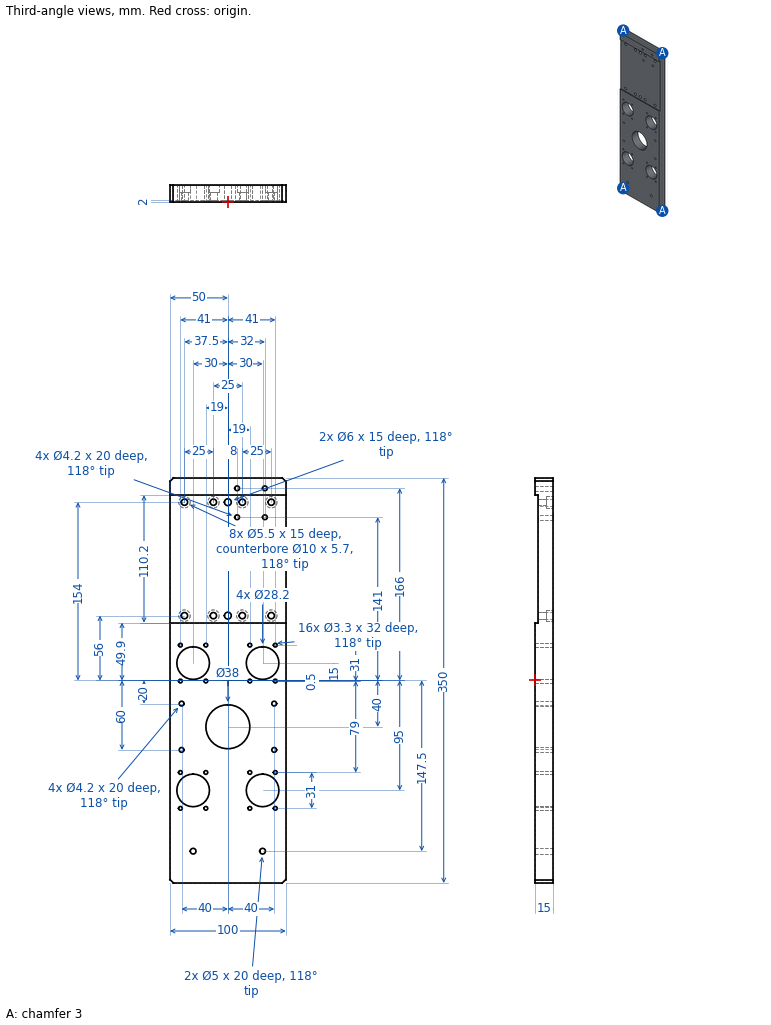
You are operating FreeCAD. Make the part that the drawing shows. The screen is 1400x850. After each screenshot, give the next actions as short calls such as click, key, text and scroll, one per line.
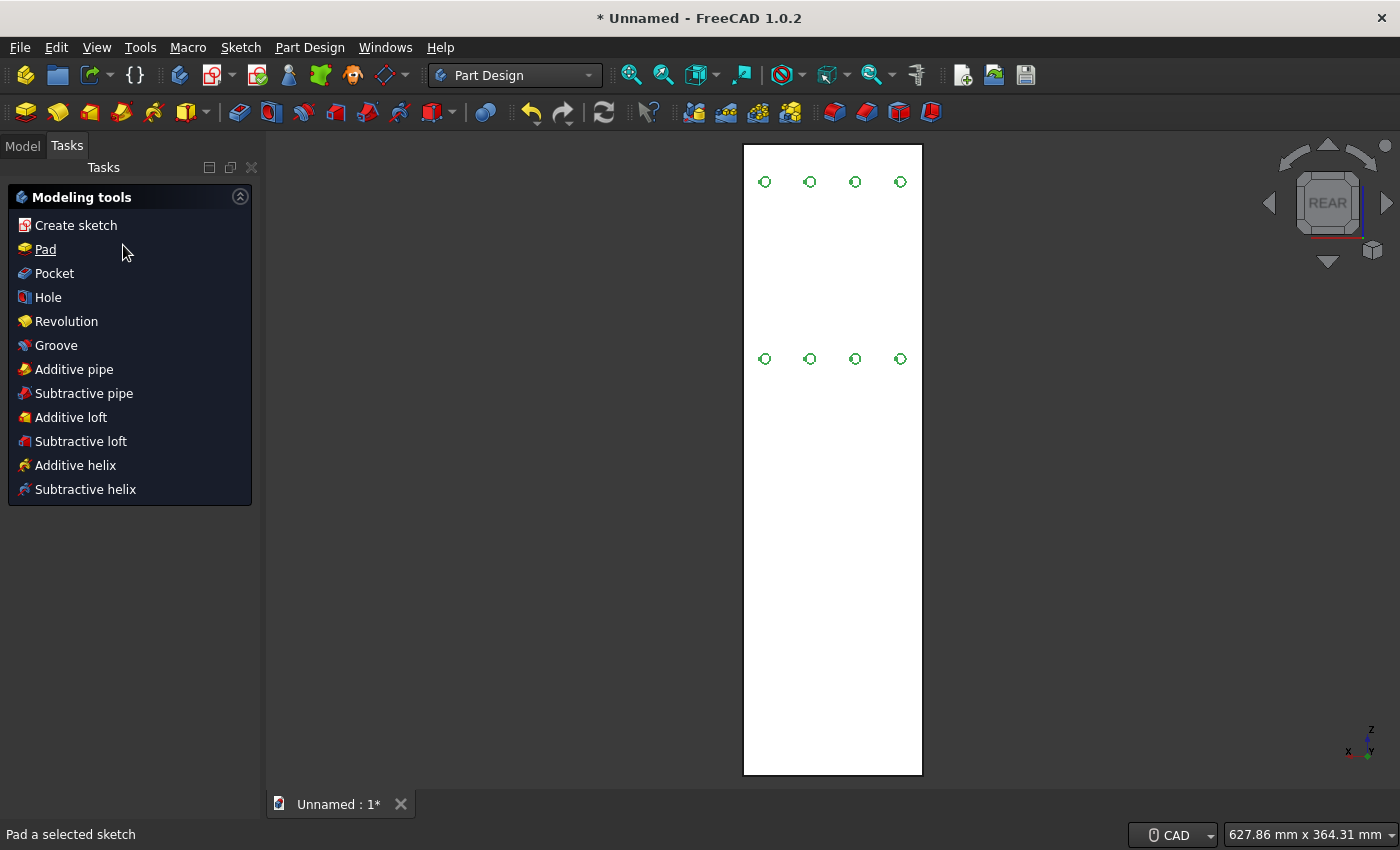
click(272, 112)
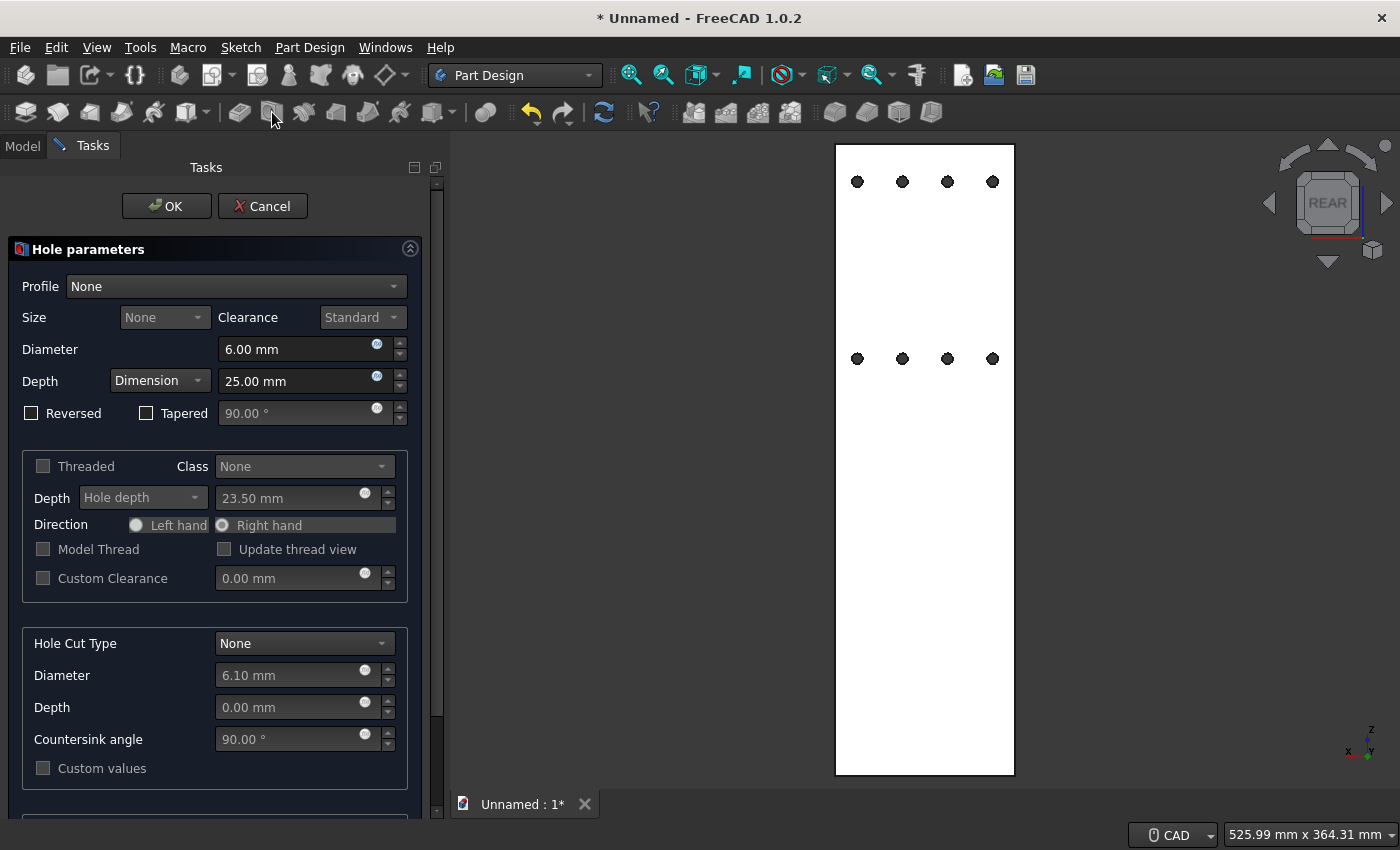
triple_click(305, 349)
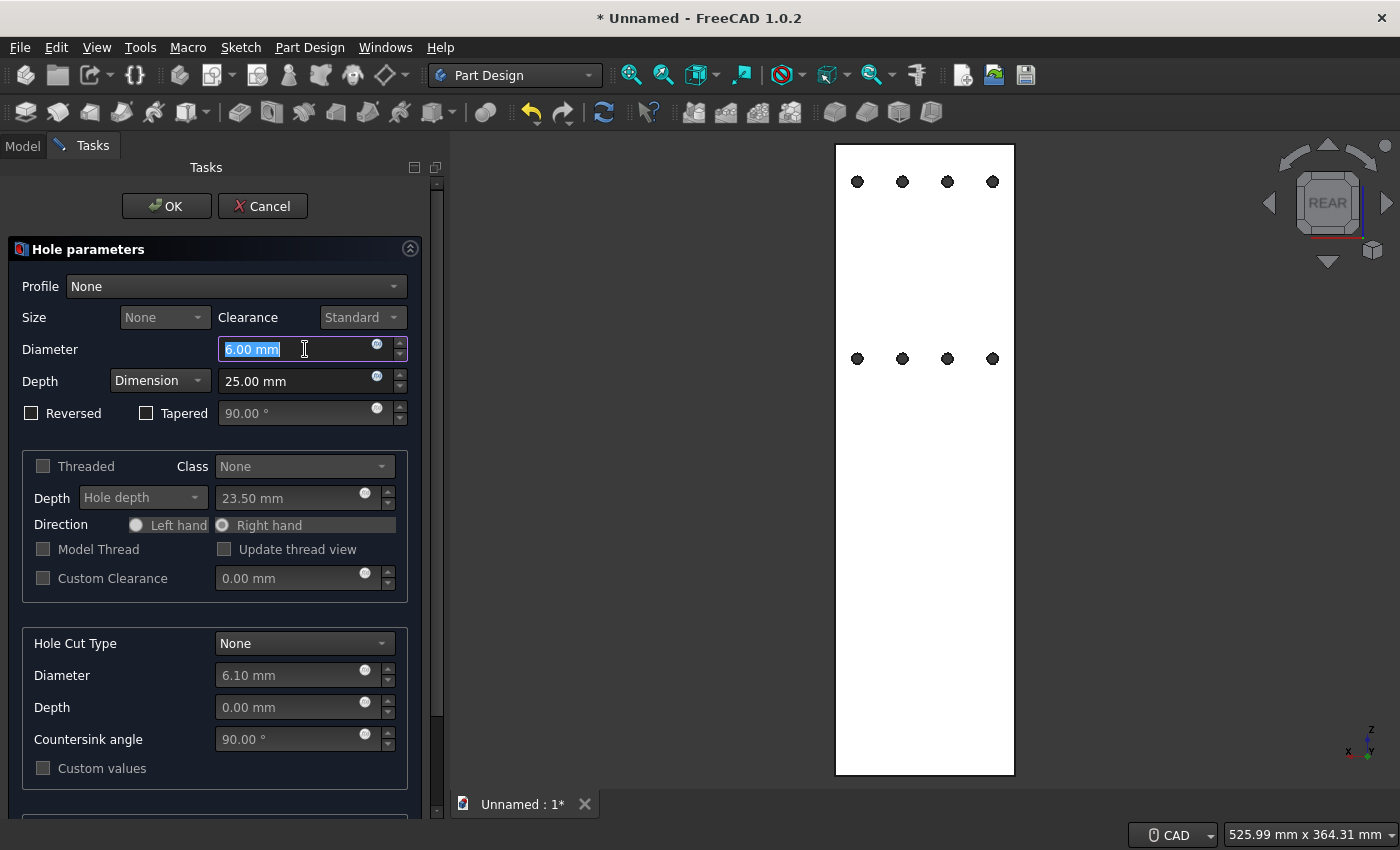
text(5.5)
key(Tab)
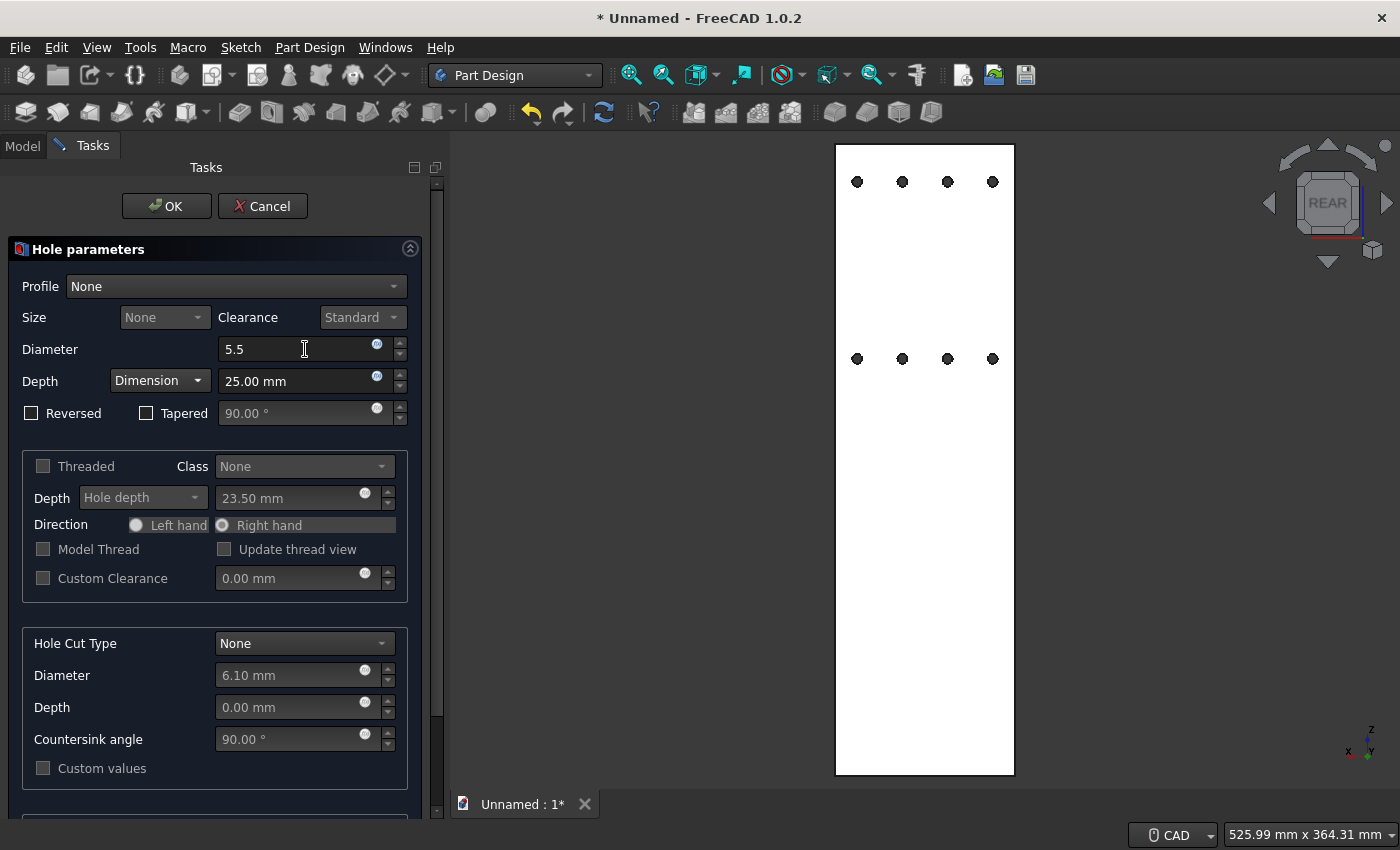
triple_click(305, 381)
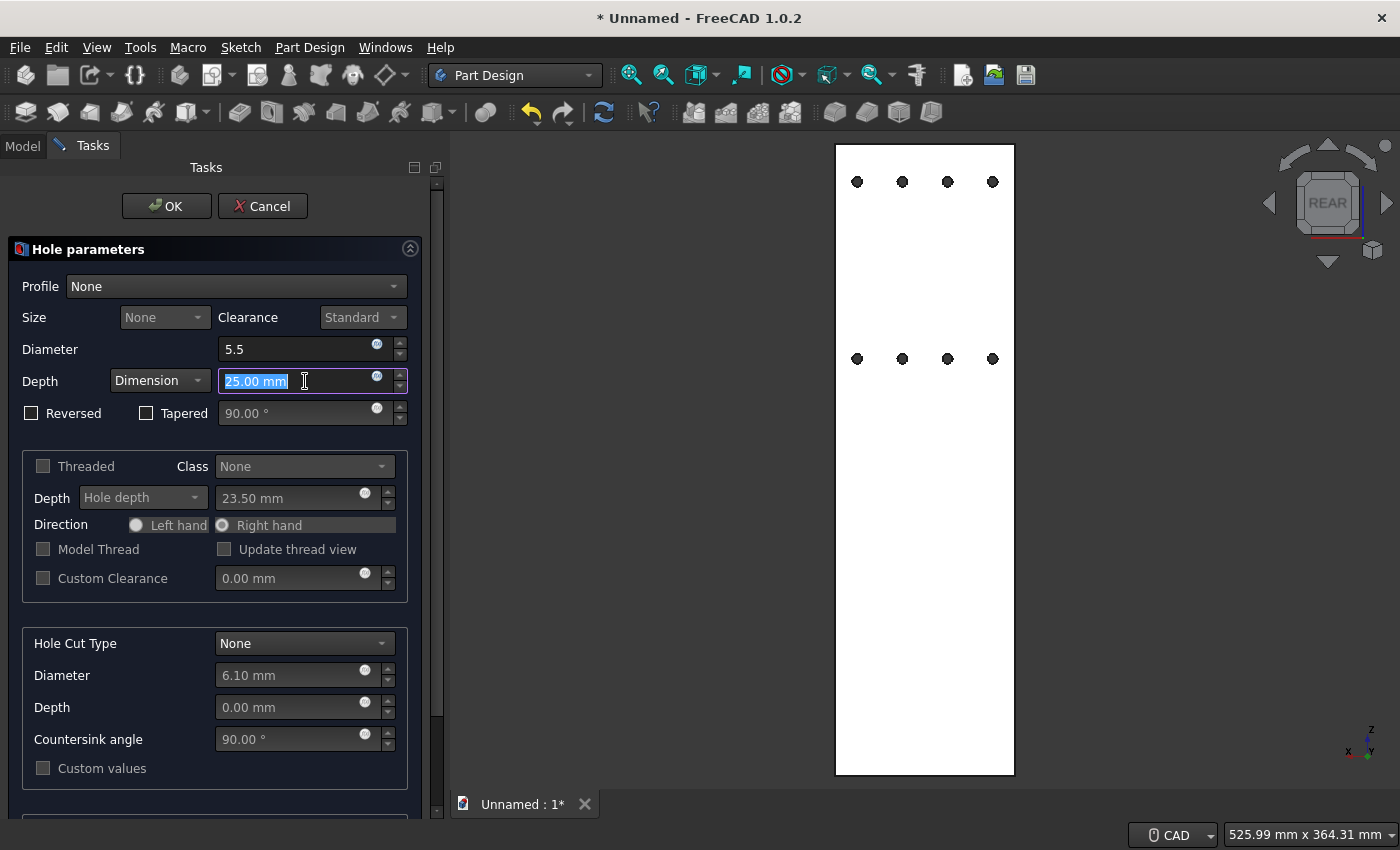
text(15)
key(Tab)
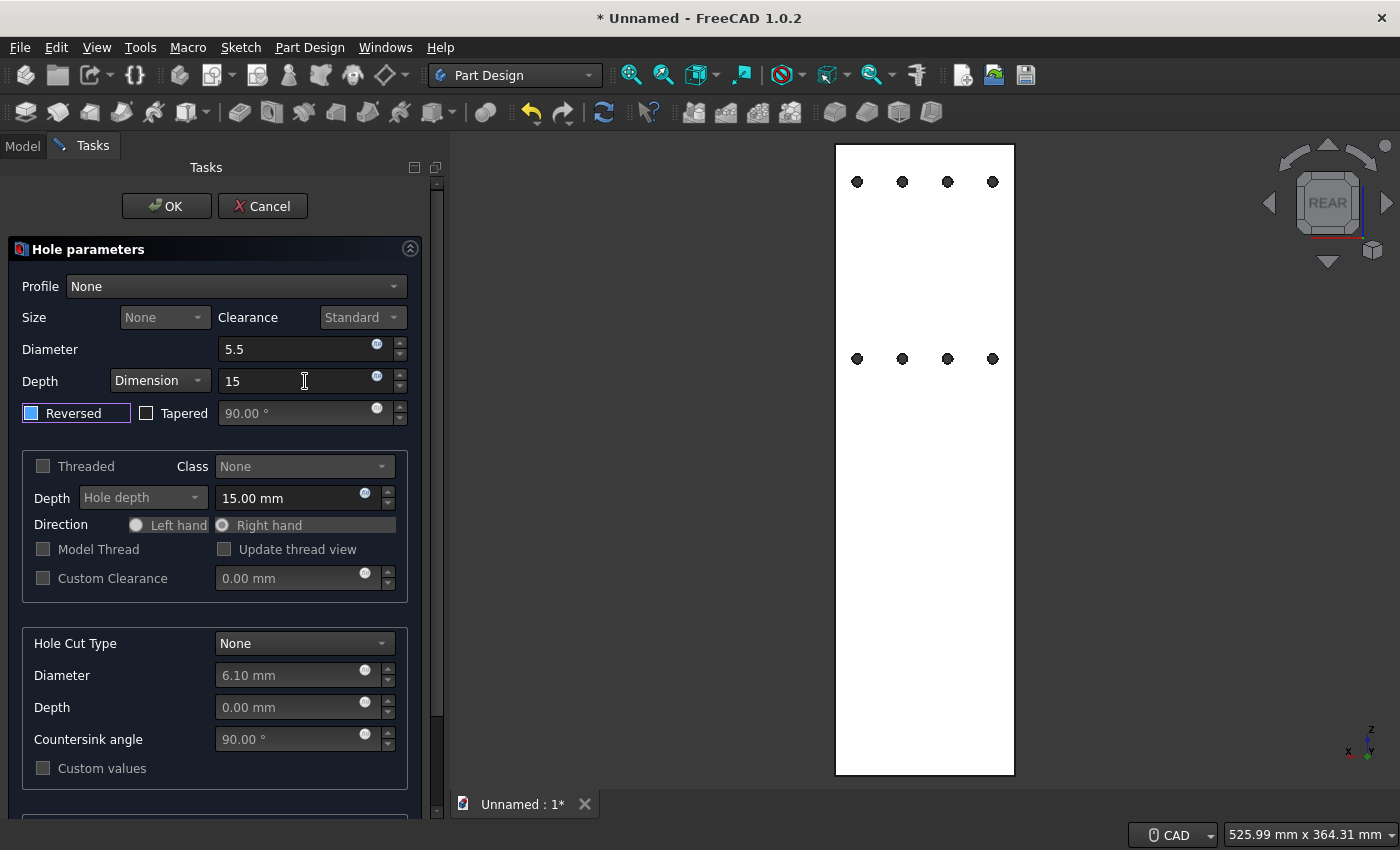
click(306, 644)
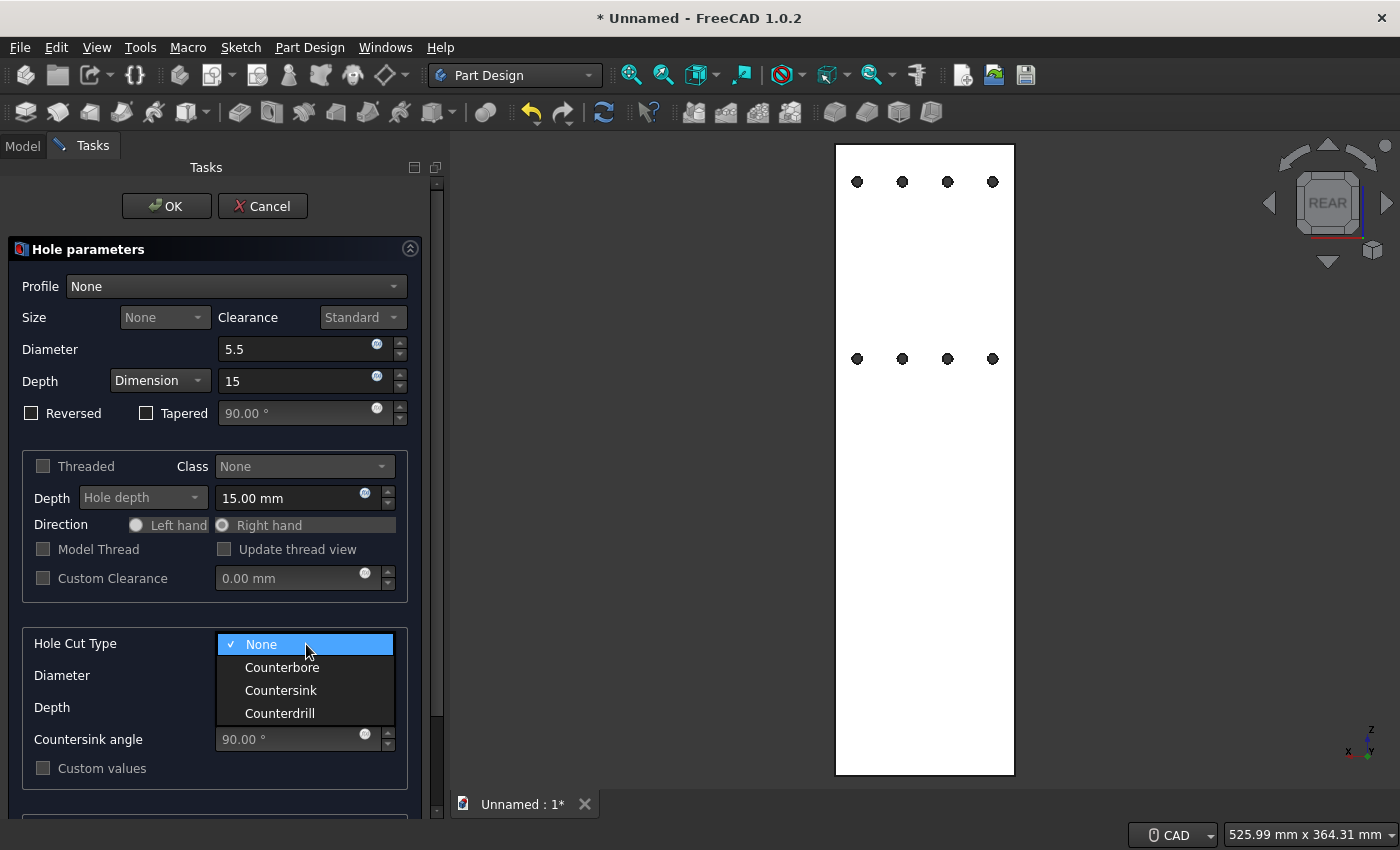
click(304, 668)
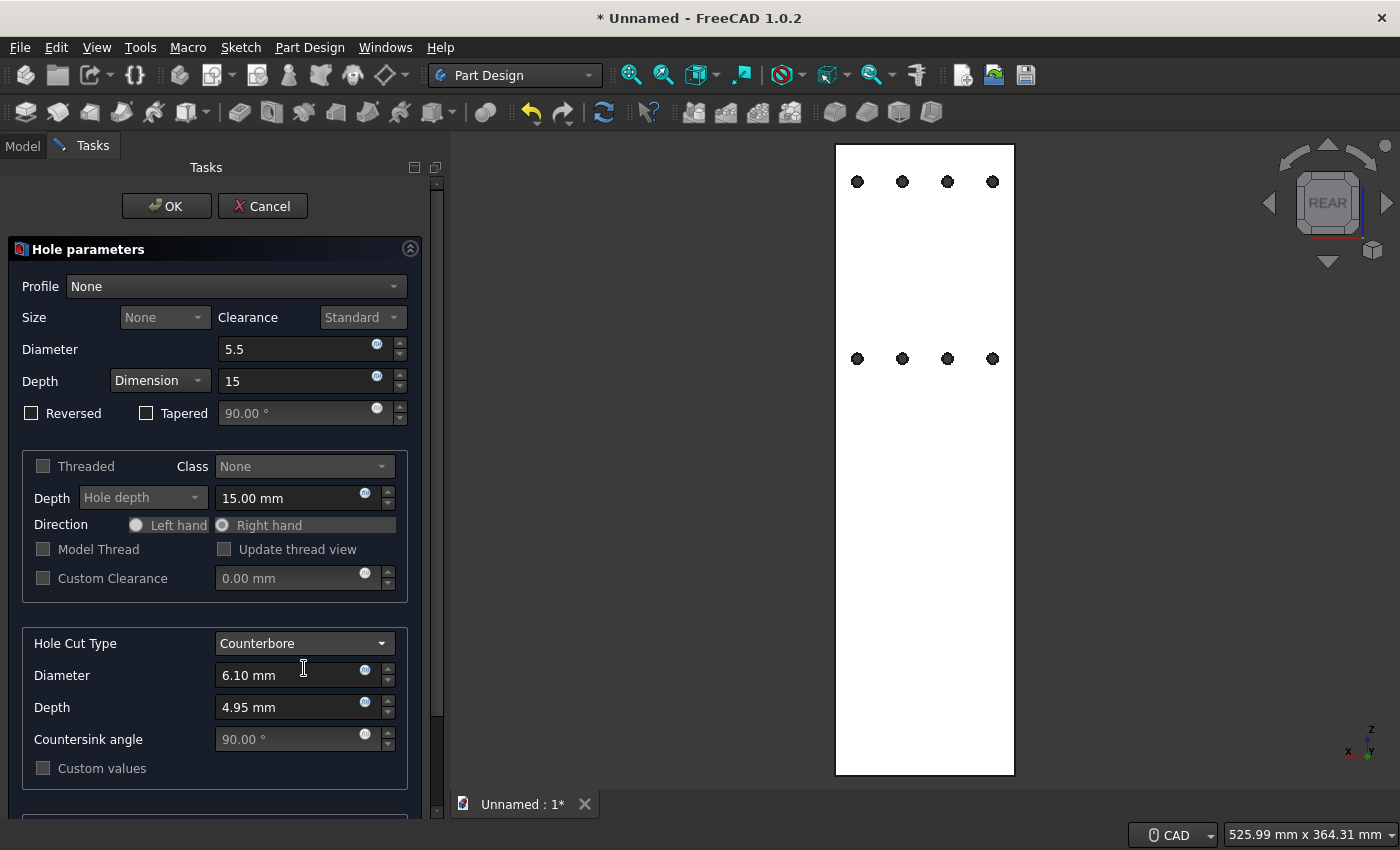
triple_click(298, 675)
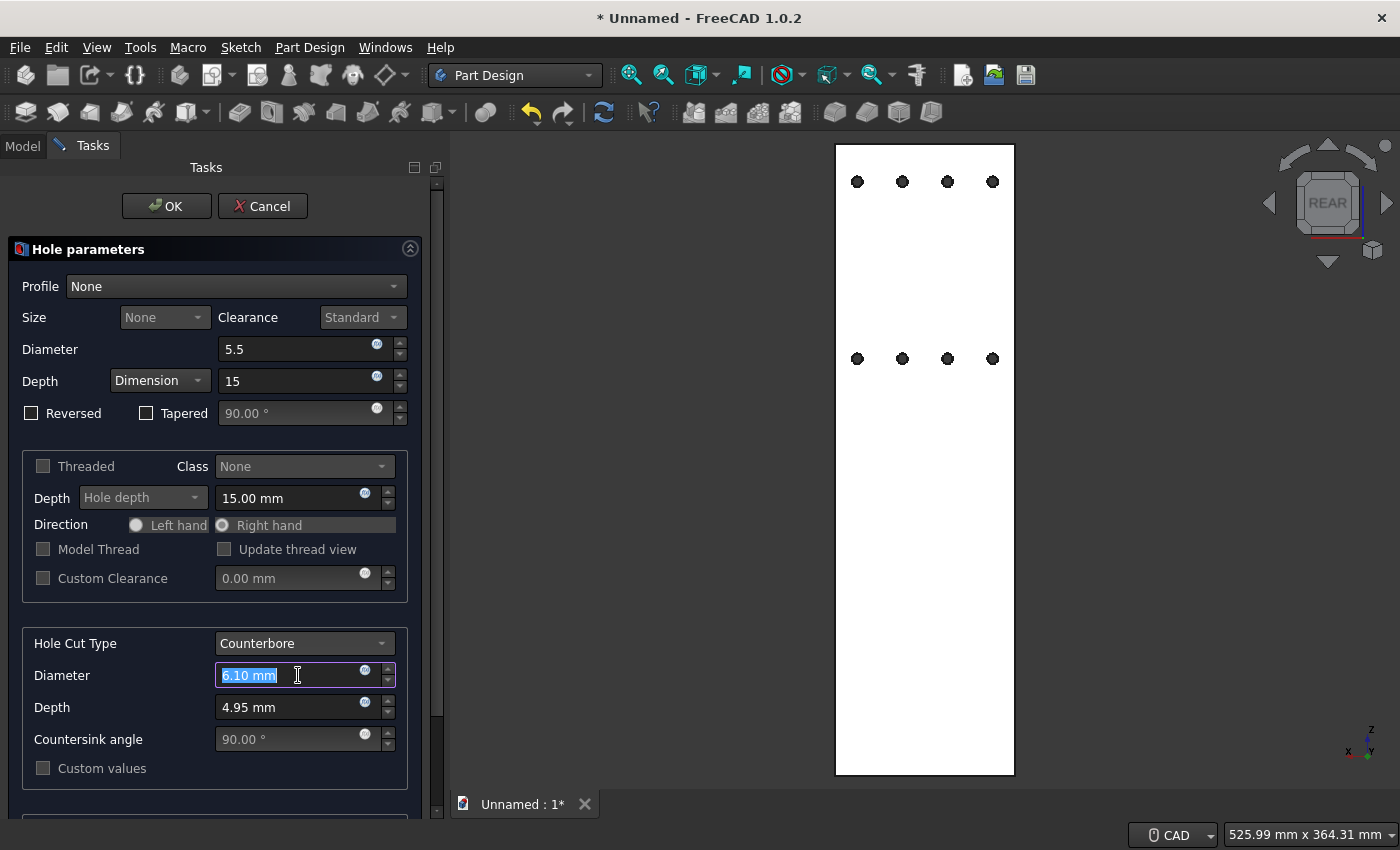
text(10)
key(Tab)